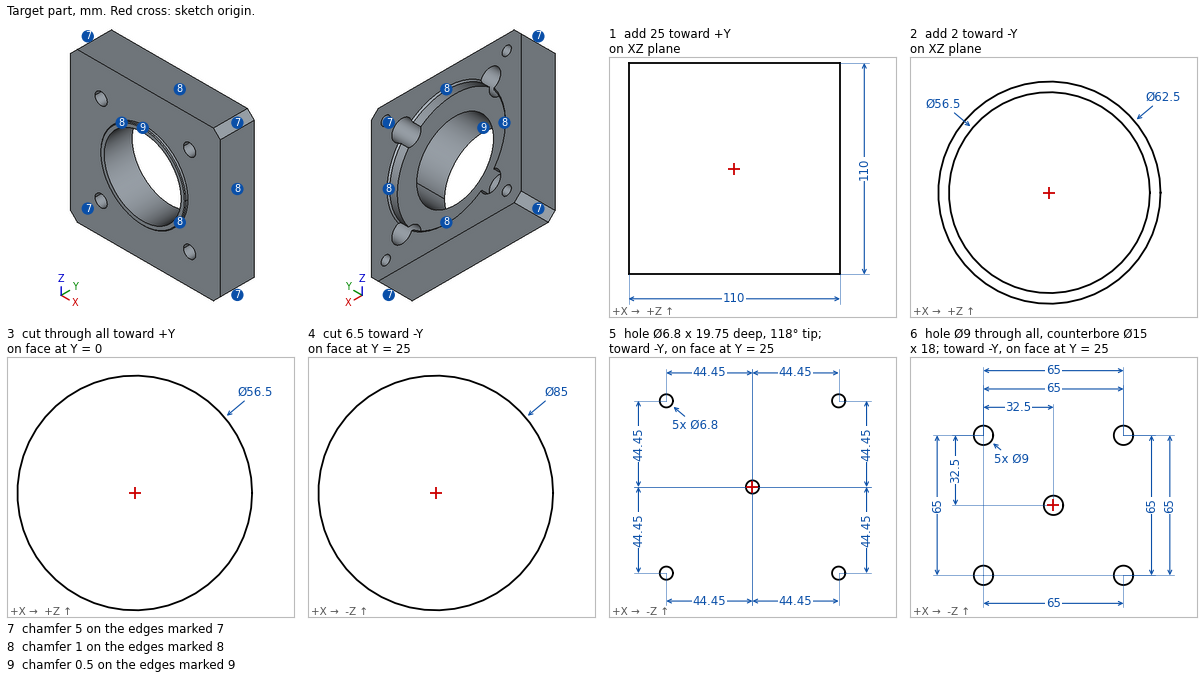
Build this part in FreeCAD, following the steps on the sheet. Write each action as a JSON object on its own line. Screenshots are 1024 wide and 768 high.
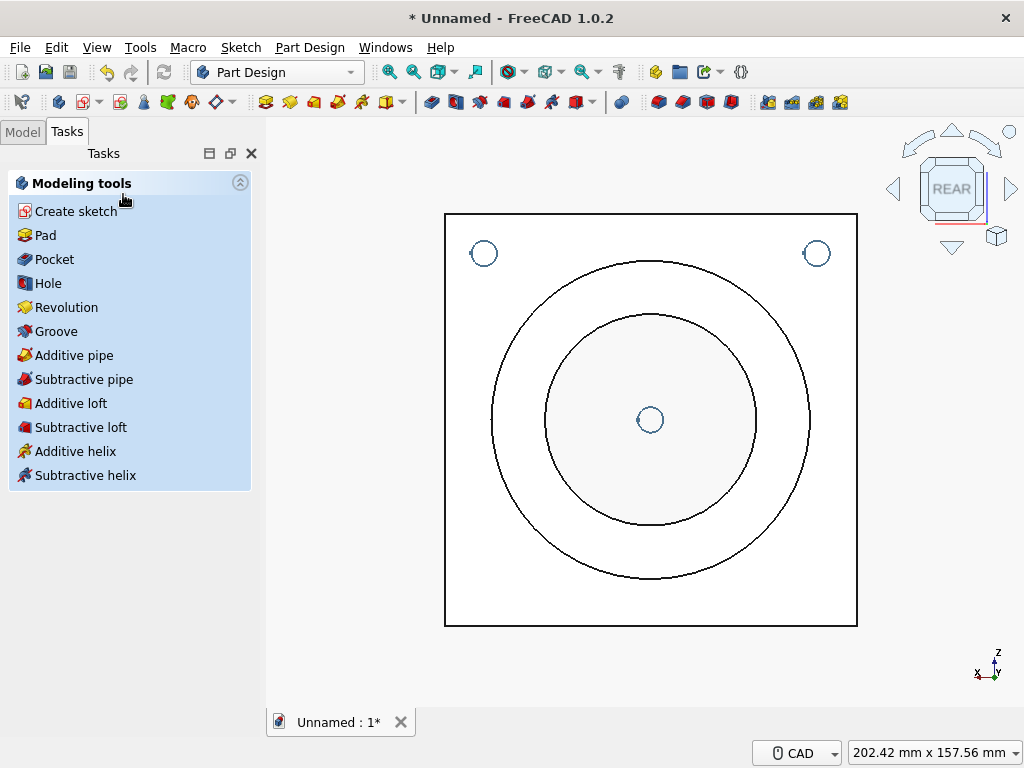
{"action": "left_click", "coordinate": [456, 102]}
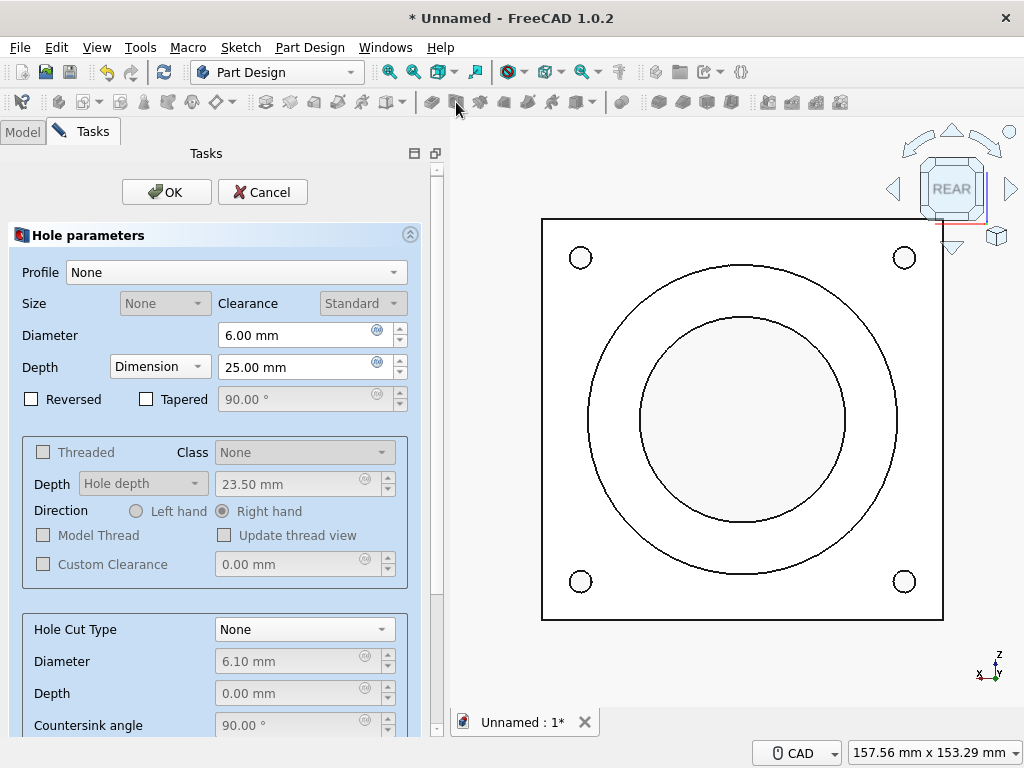
{"action": "triple_click", "coordinate": [305, 335]}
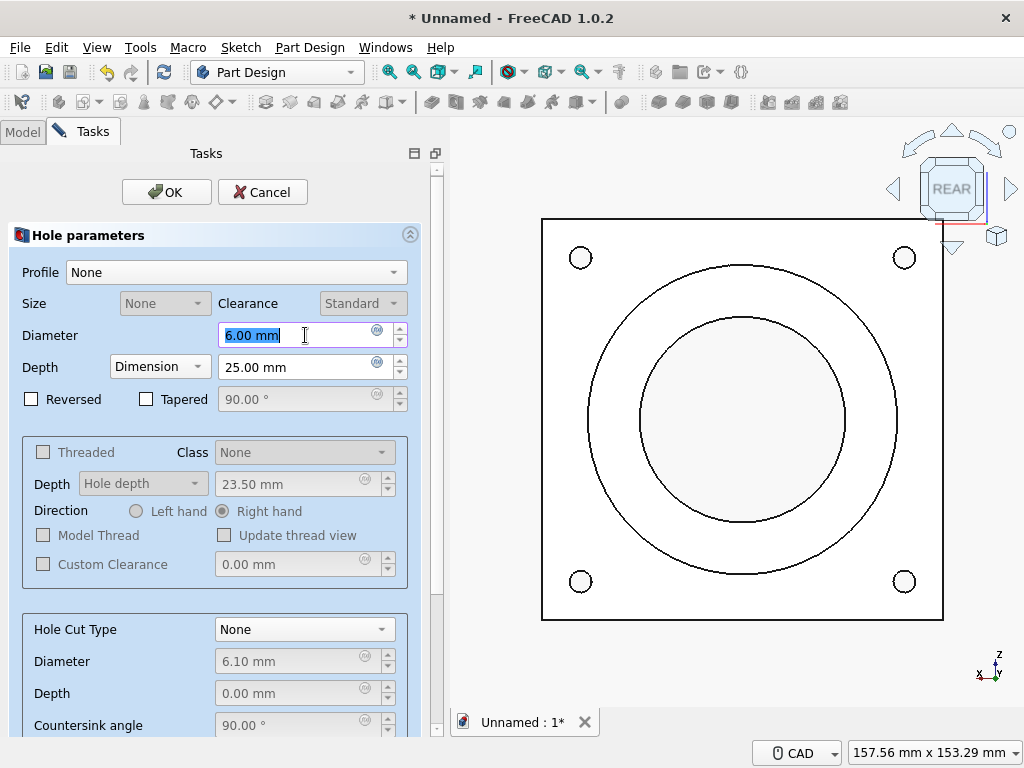
{"action": "type", "text": "6.8"}
{"action": "key", "text": "Tab"}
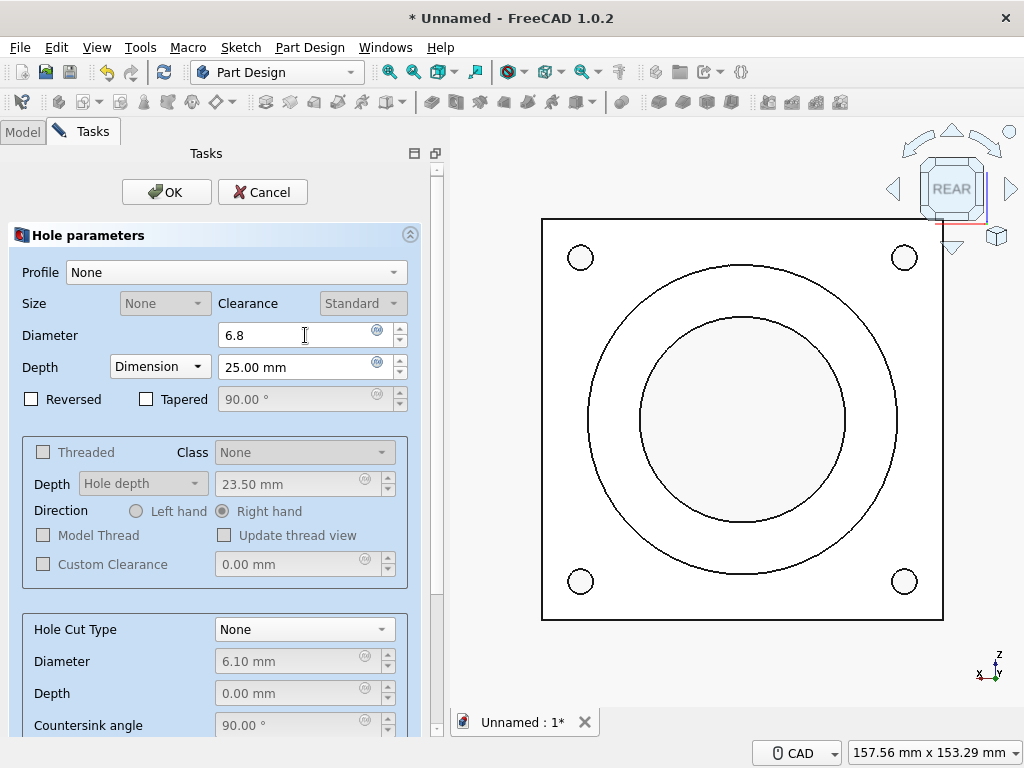
{"action": "triple_click", "coordinate": [305, 367]}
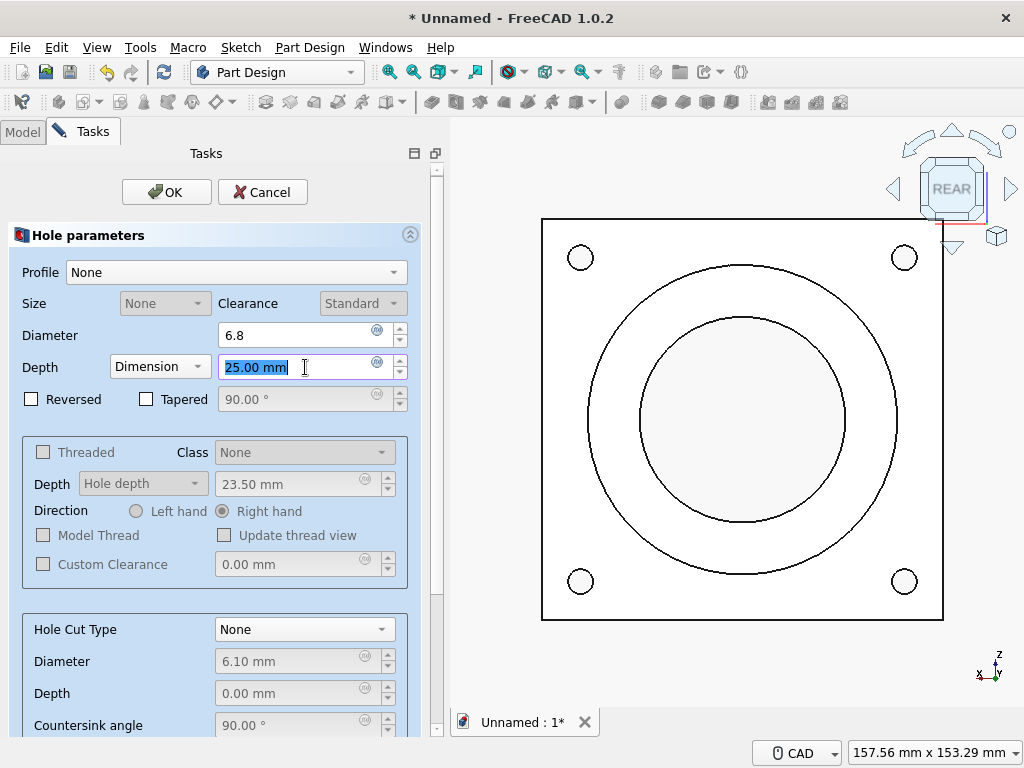
{"action": "type", "text": "19.75"}
{"action": "key", "text": "Tab"}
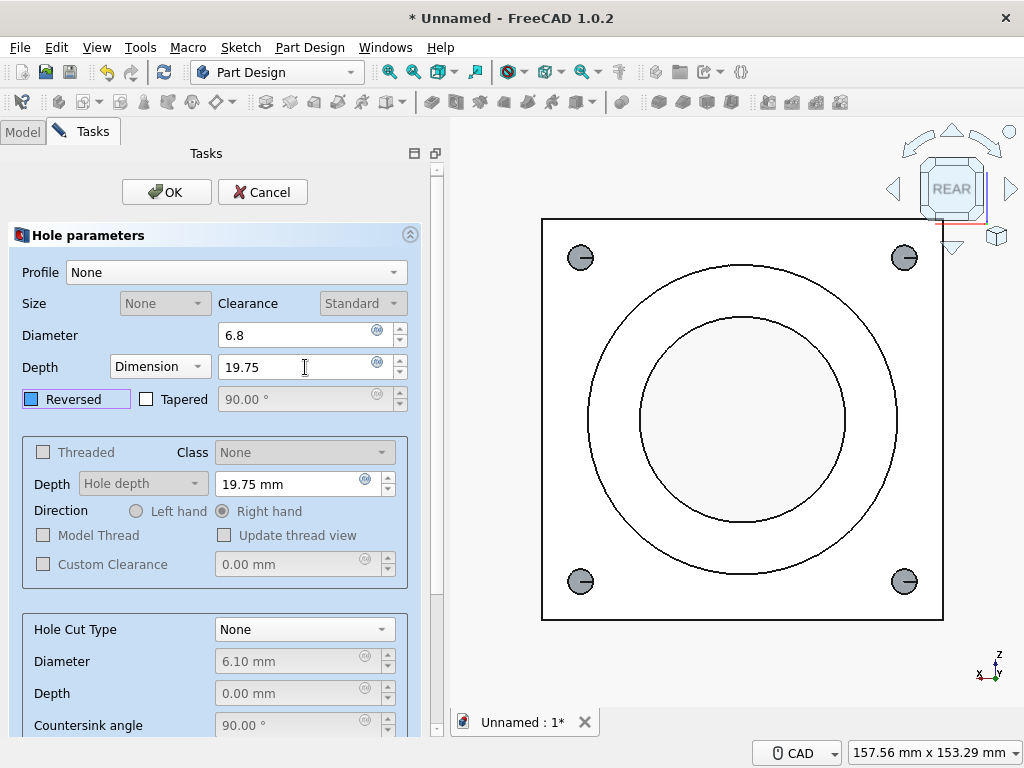
{"action": "left_click", "coordinate": [167, 192]}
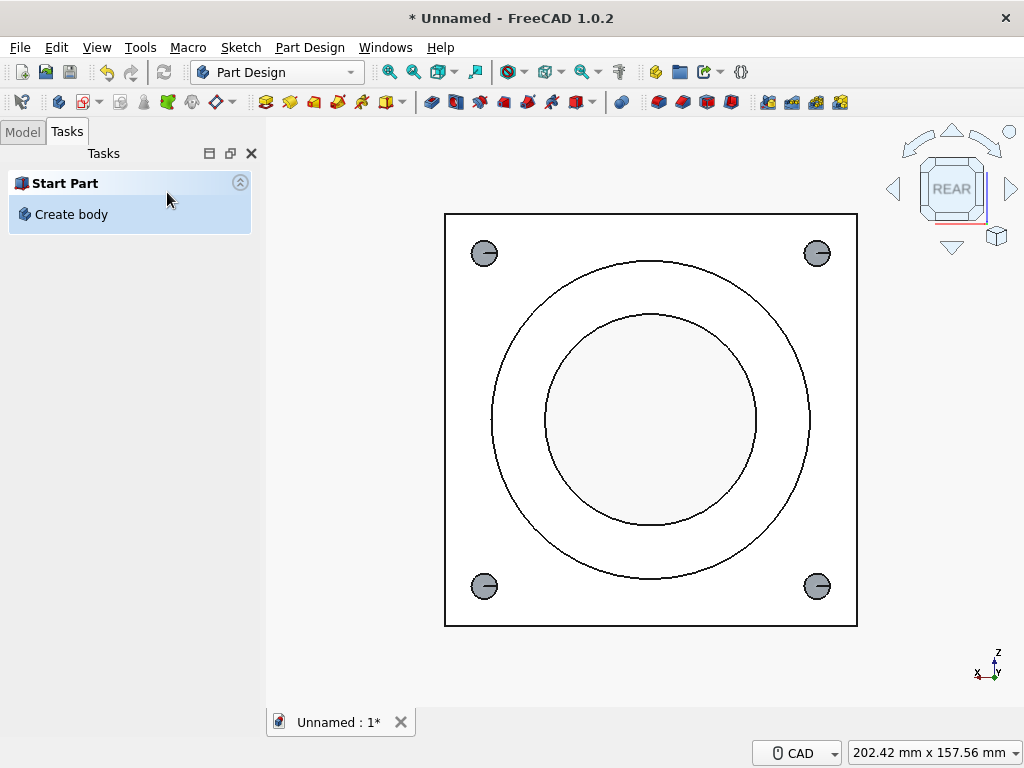
{"action": "left_click", "coordinate": [474, 301]}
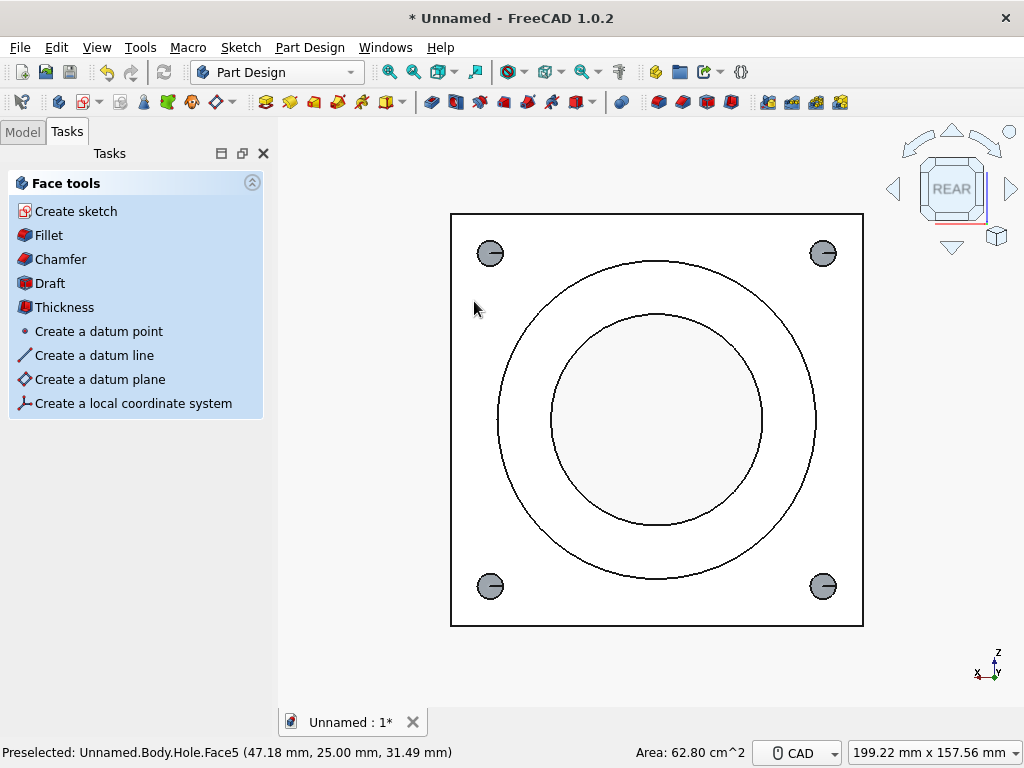
{"action": "left_click", "coordinate": [84, 102]}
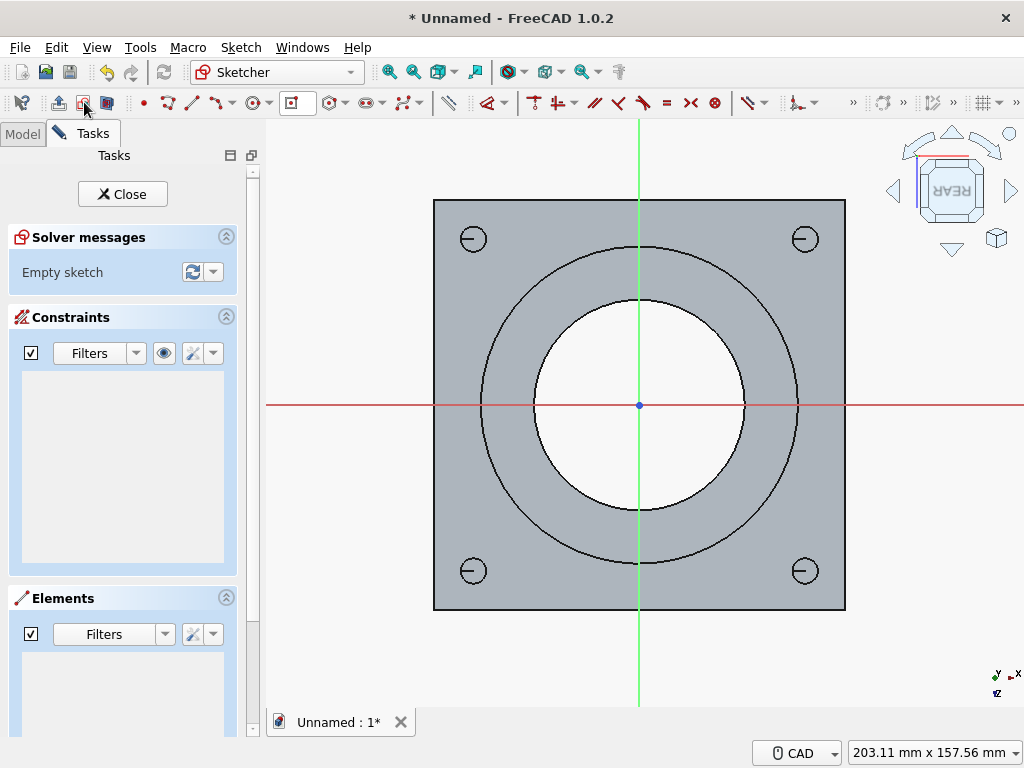
{"action": "scroll", "coordinate": [767, 389], "scroll_direction": "up", "scroll_amount": 2}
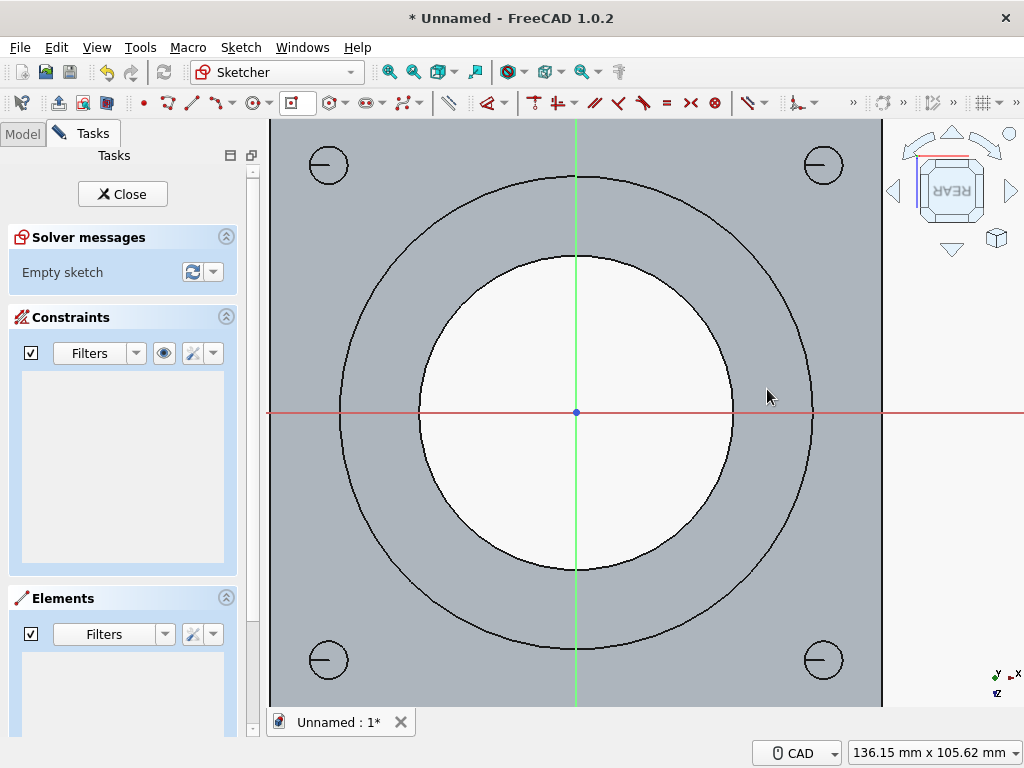
{"action": "left_click", "coordinate": [254, 104]}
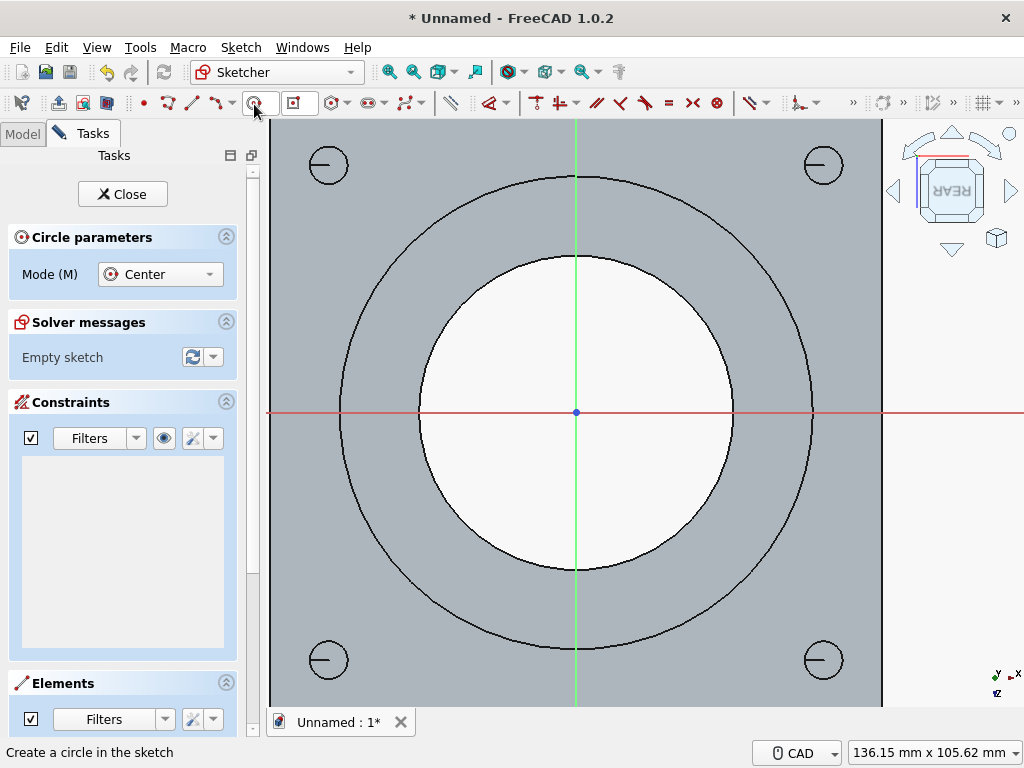
{"action": "left_click", "coordinate": [395, 232]}
{"action": "left_click", "coordinate": [413, 214]}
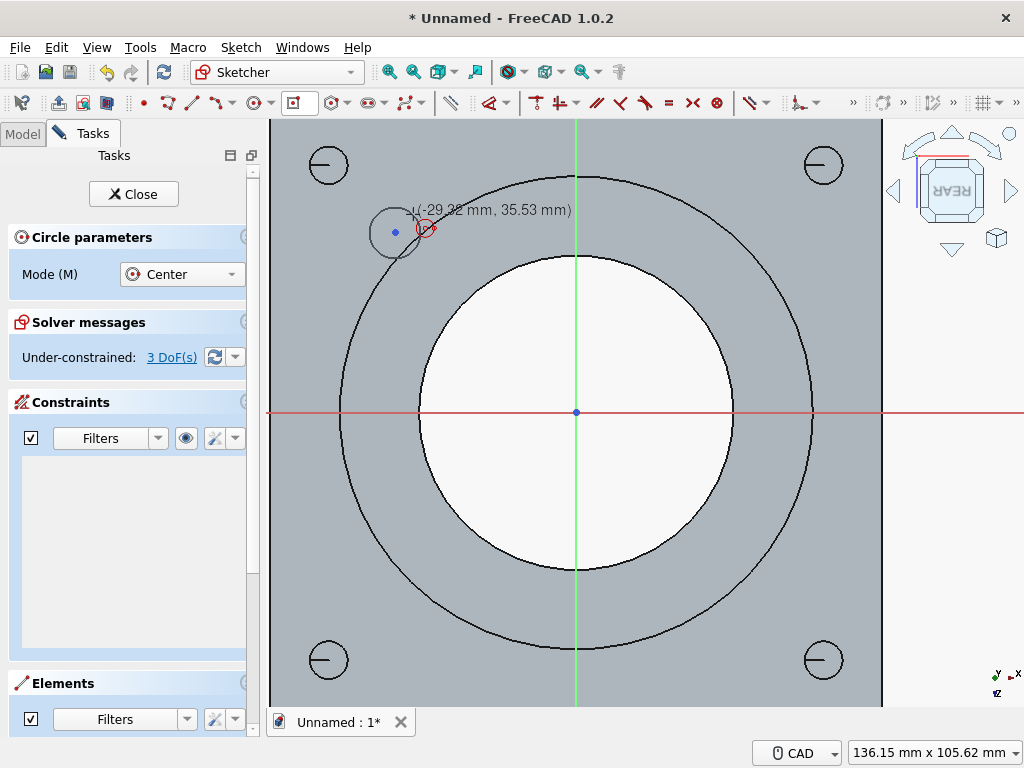
{"action": "left_click", "coordinate": [576, 413]}
{"action": "left_click", "coordinate": [594, 395]}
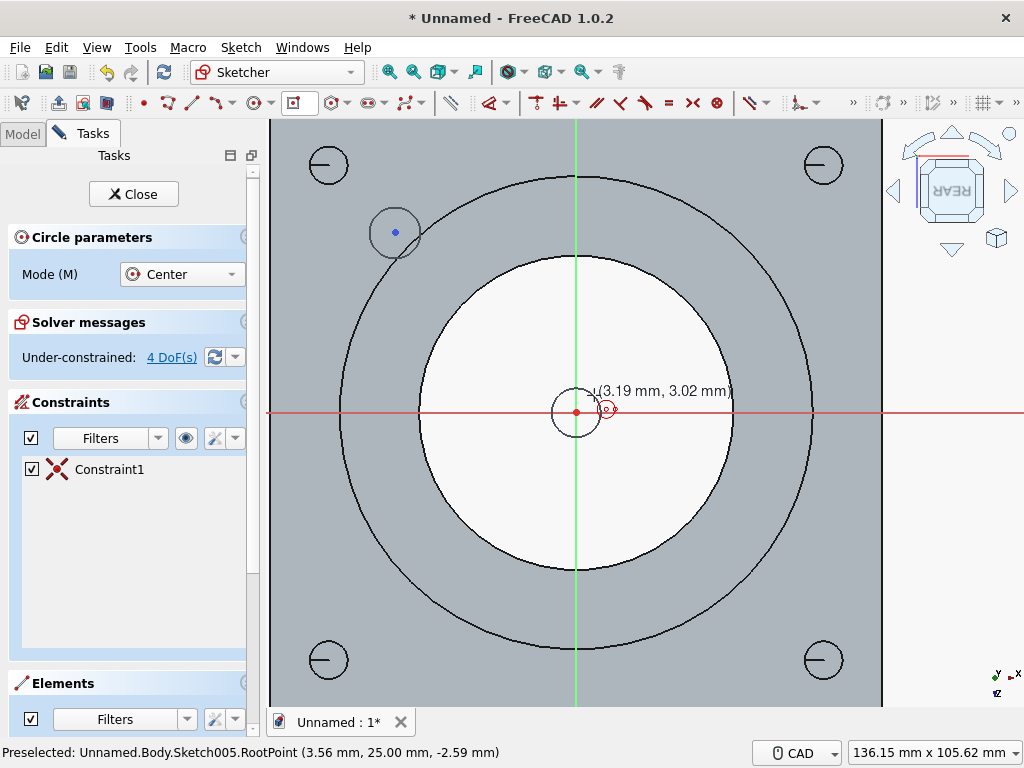
{"action": "left_click", "coordinate": [757, 232]}
{"action": "left_click", "coordinate": [775, 214]}